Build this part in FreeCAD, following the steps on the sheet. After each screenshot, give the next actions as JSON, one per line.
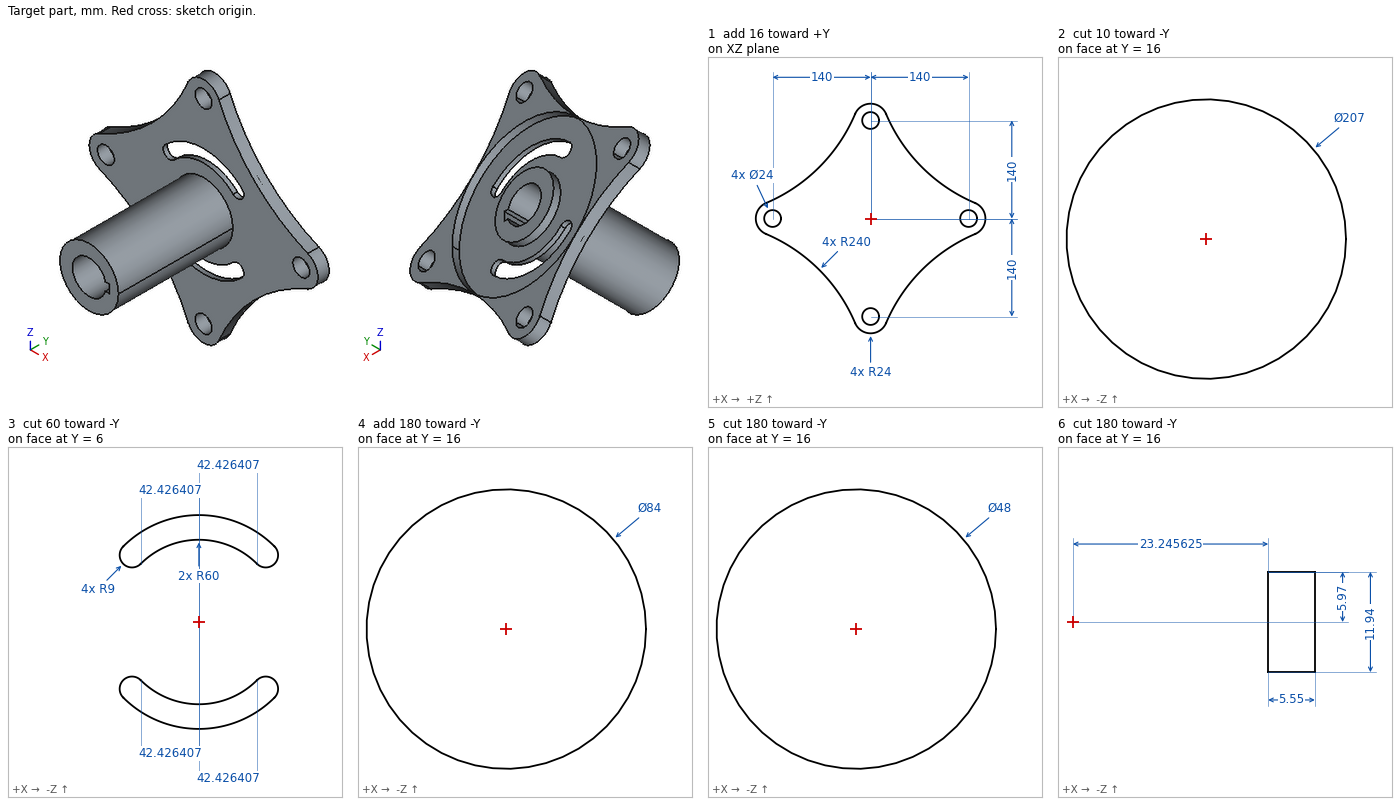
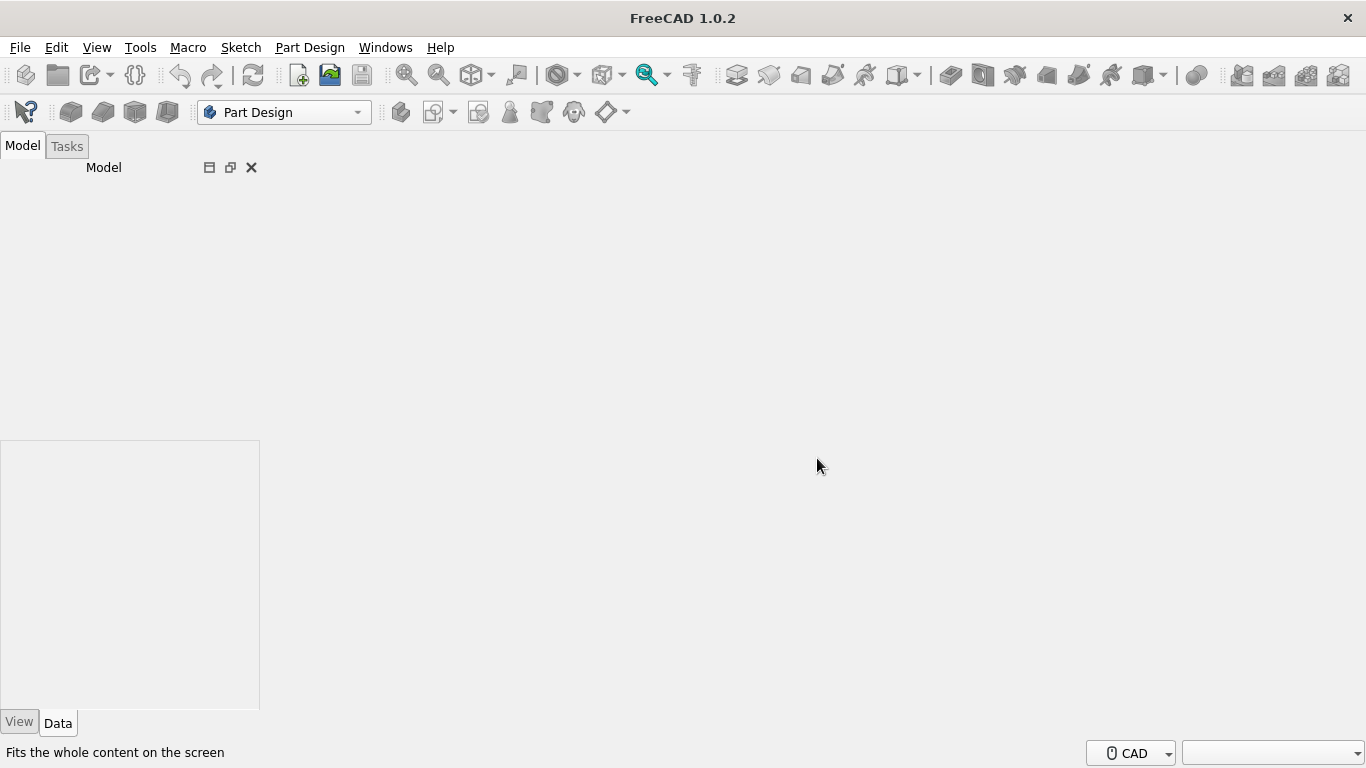
{"action": "left_click", "coordinate": [298, 76]}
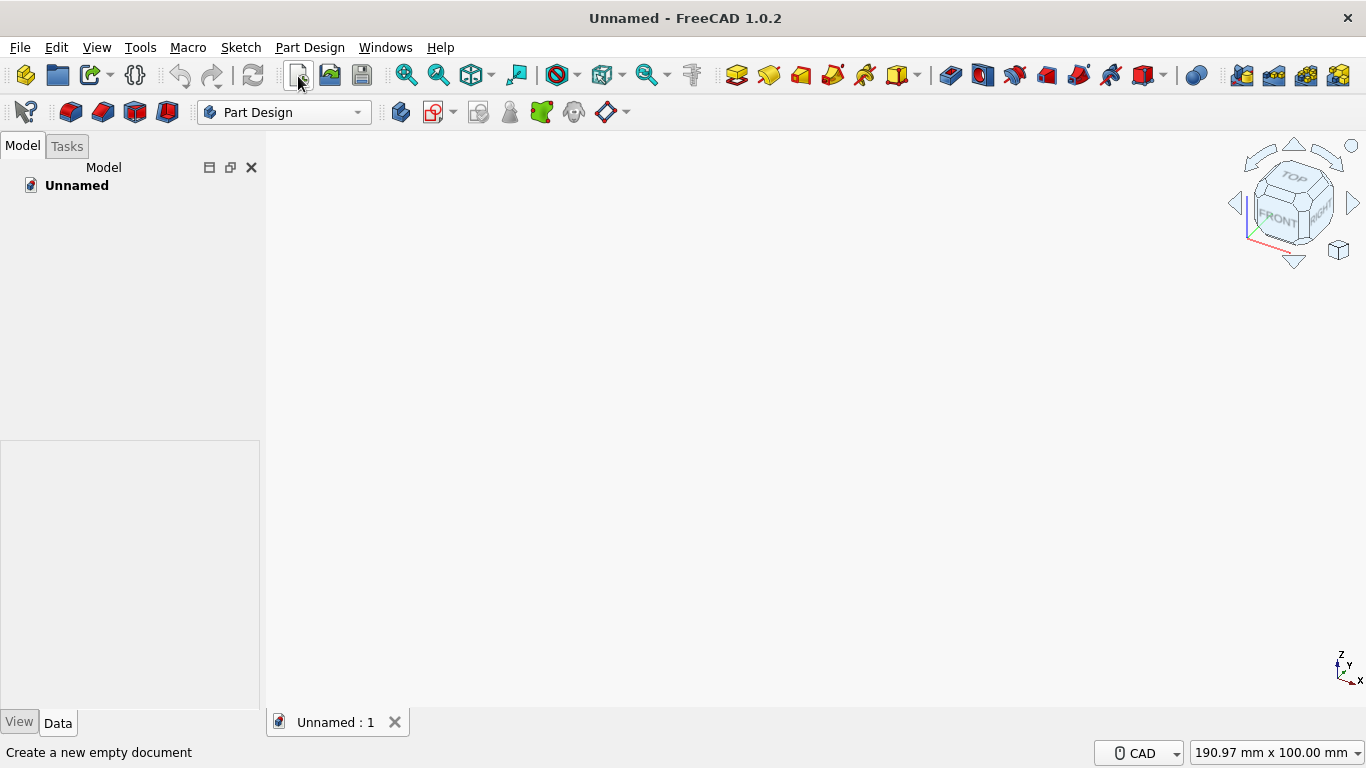
{"action": "left_click", "coordinate": [434, 112]}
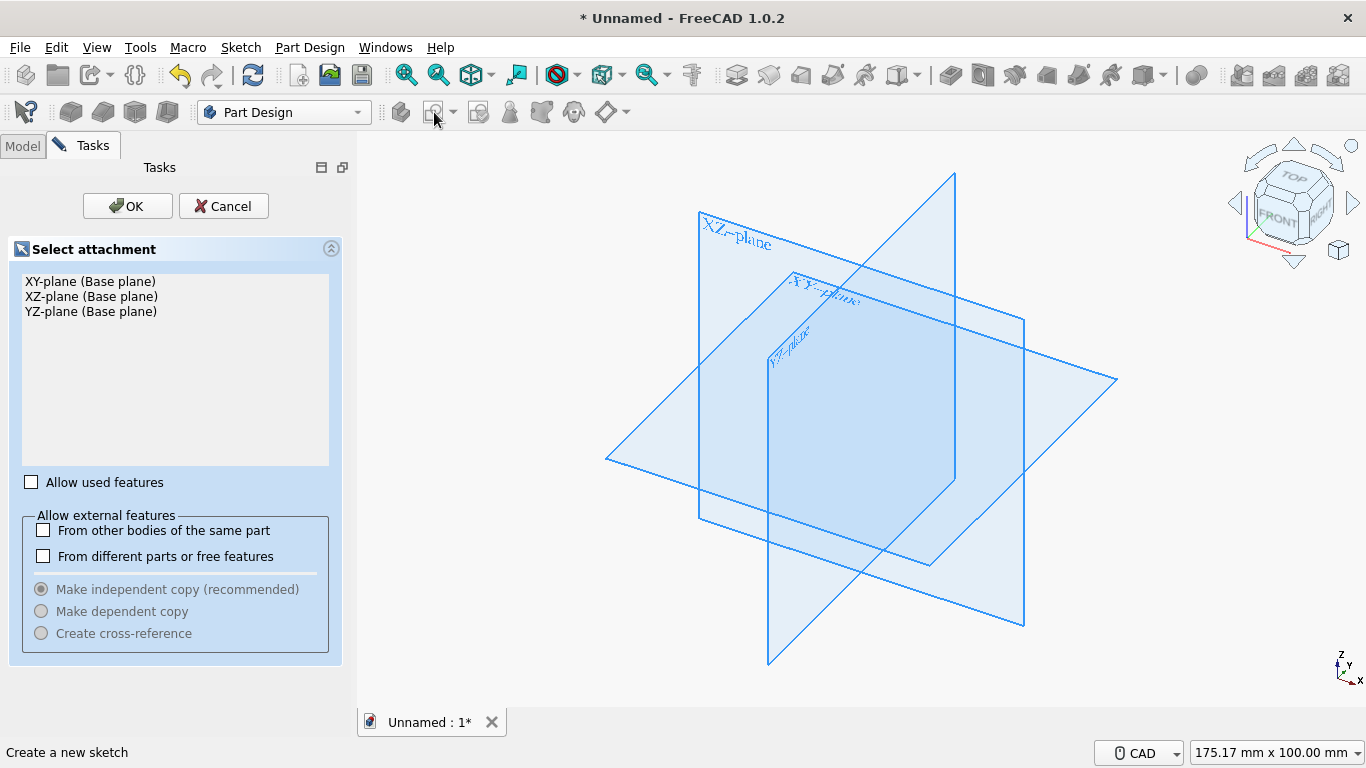
{"action": "left_click", "coordinate": [82, 296]}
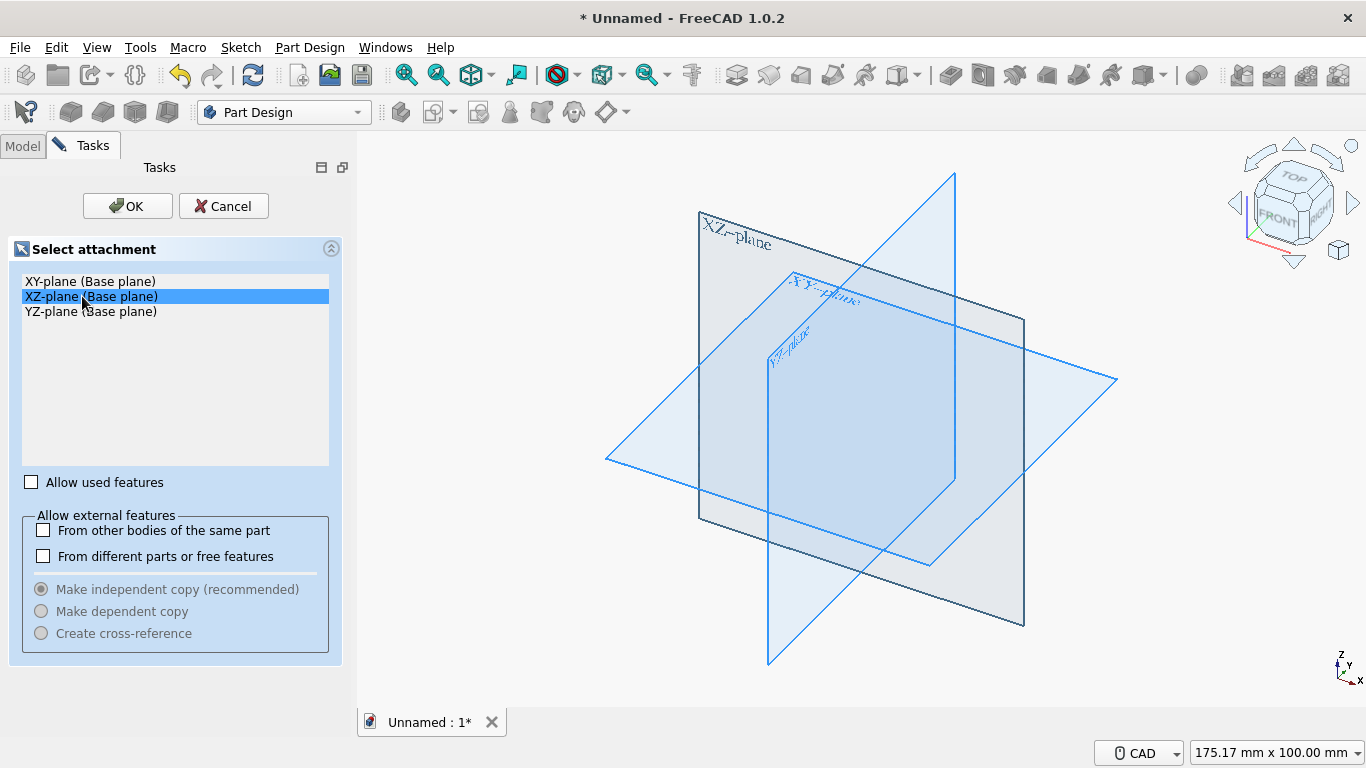
{"action": "left_click", "coordinate": [128, 206]}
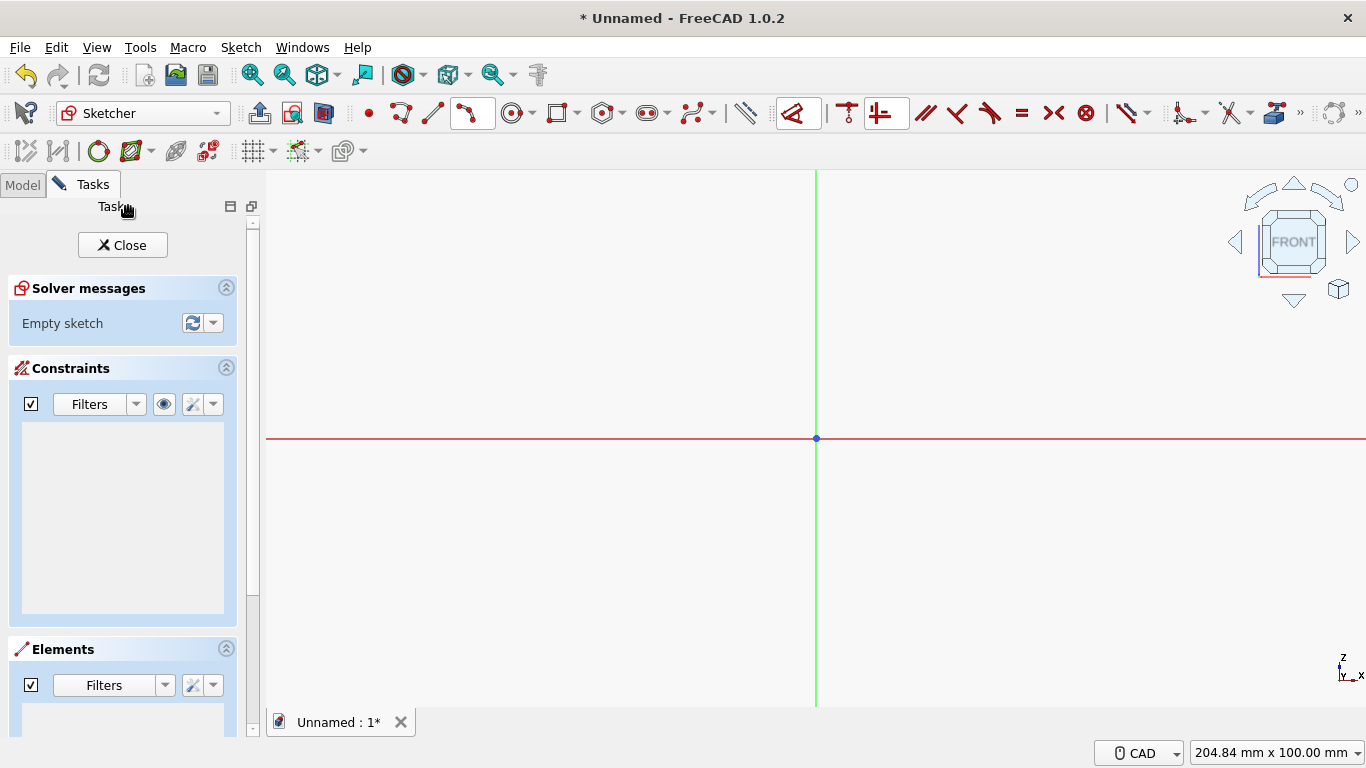
{"action": "scroll", "coordinate": [730, 438], "scroll_direction": "down", "scroll_amount": 8}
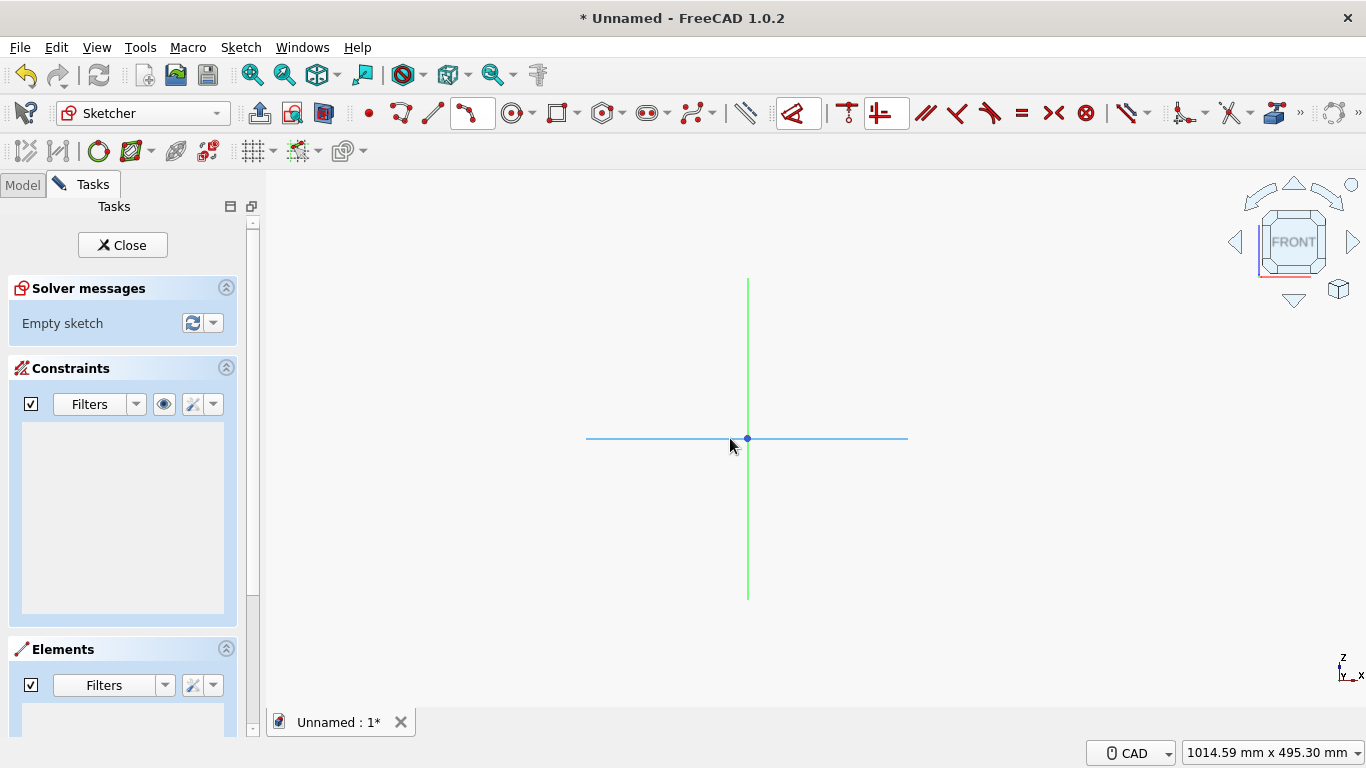
{"action": "left_click", "coordinate": [466, 114]}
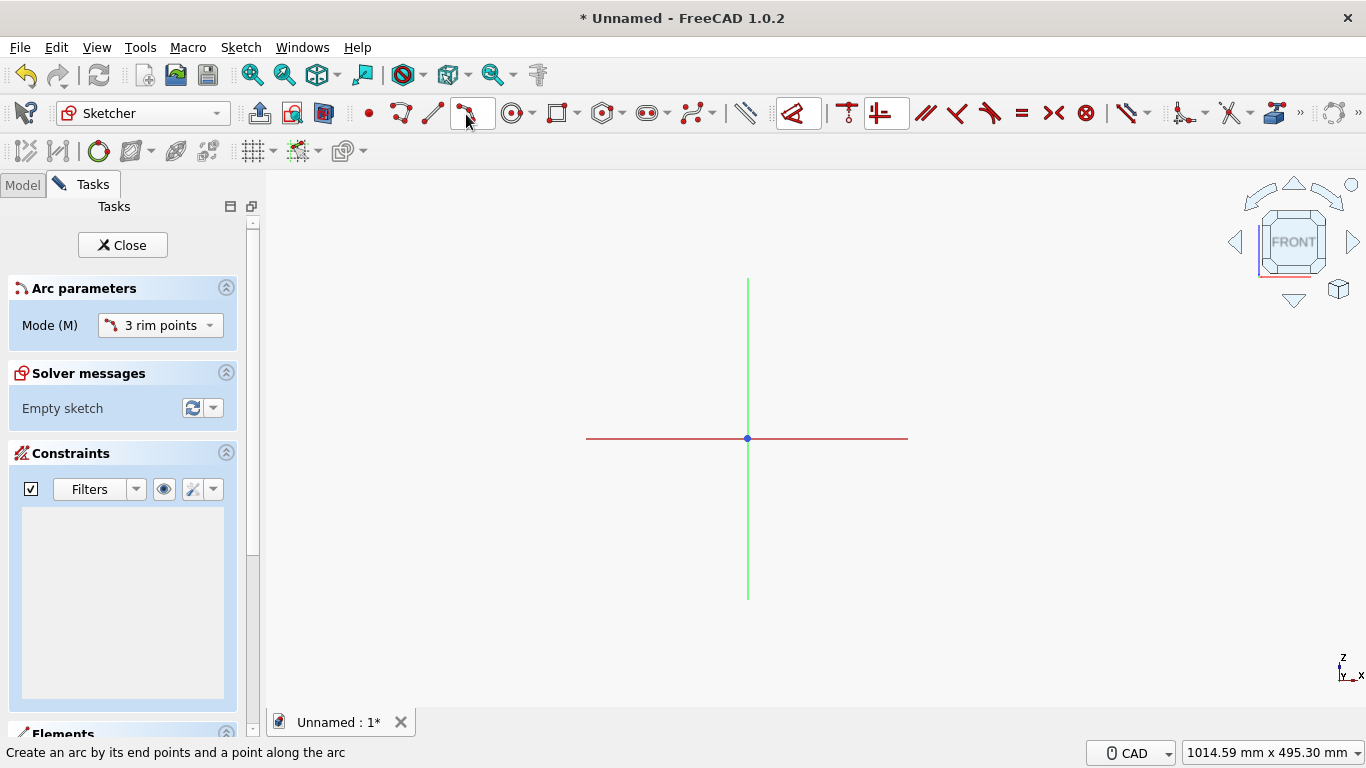
{"action": "left_click", "coordinate": [772, 600]}
{"action": "left_click", "coordinate": [724, 600]}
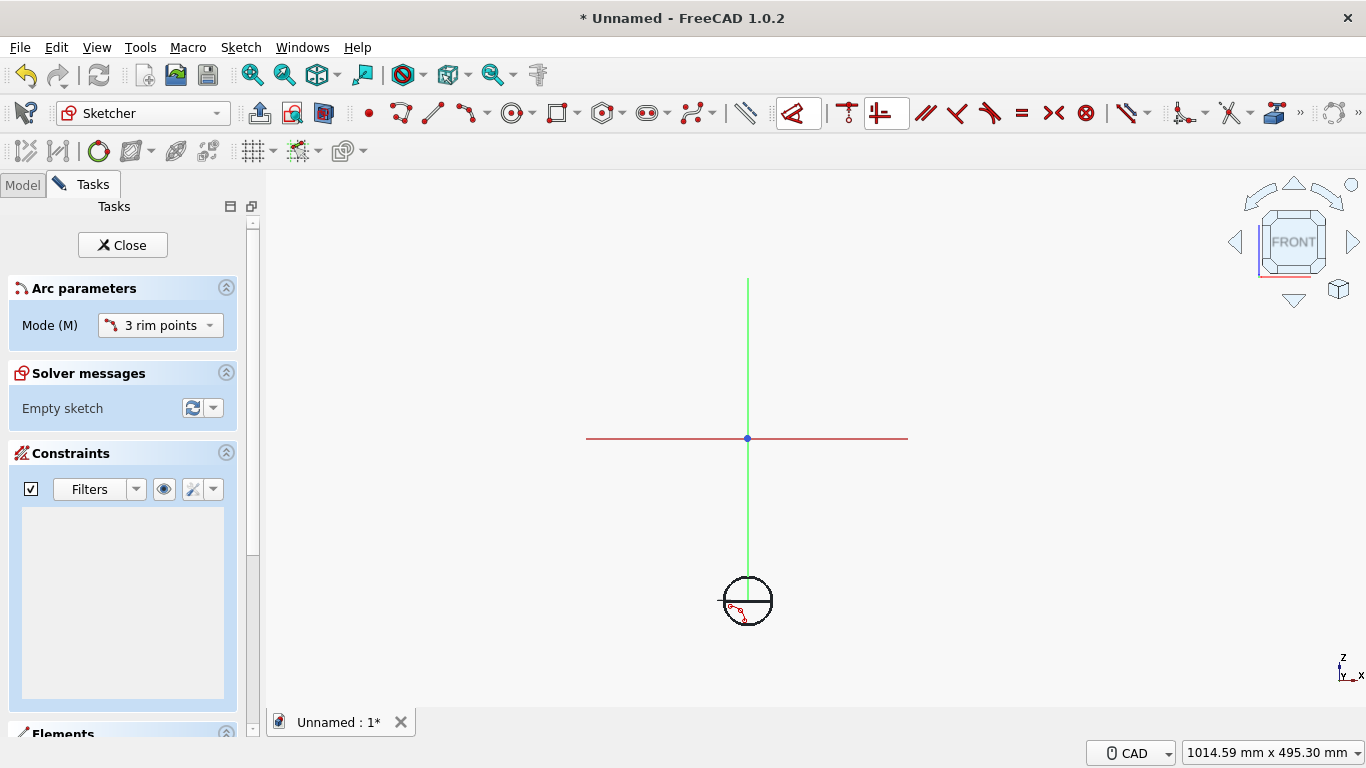
{"action": "scroll", "coordinate": [736, 614], "scroll_direction": "up", "scroll_amount": 2}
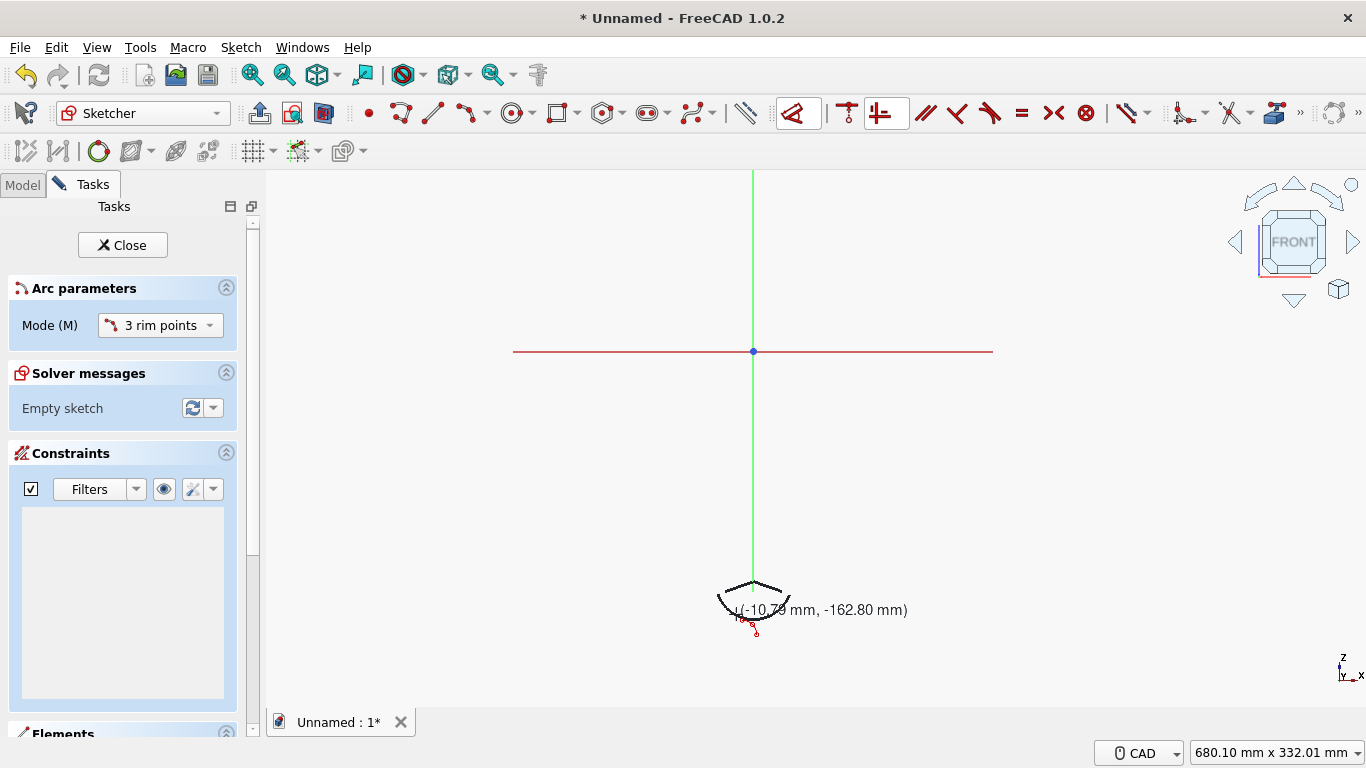
{"action": "left_click", "coordinate": [736, 613]}